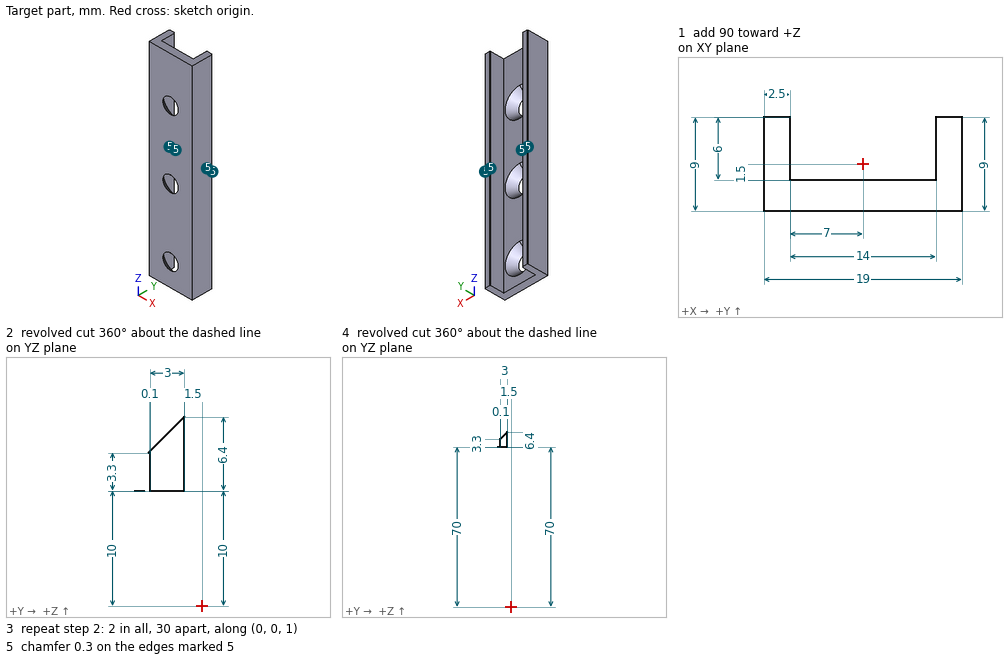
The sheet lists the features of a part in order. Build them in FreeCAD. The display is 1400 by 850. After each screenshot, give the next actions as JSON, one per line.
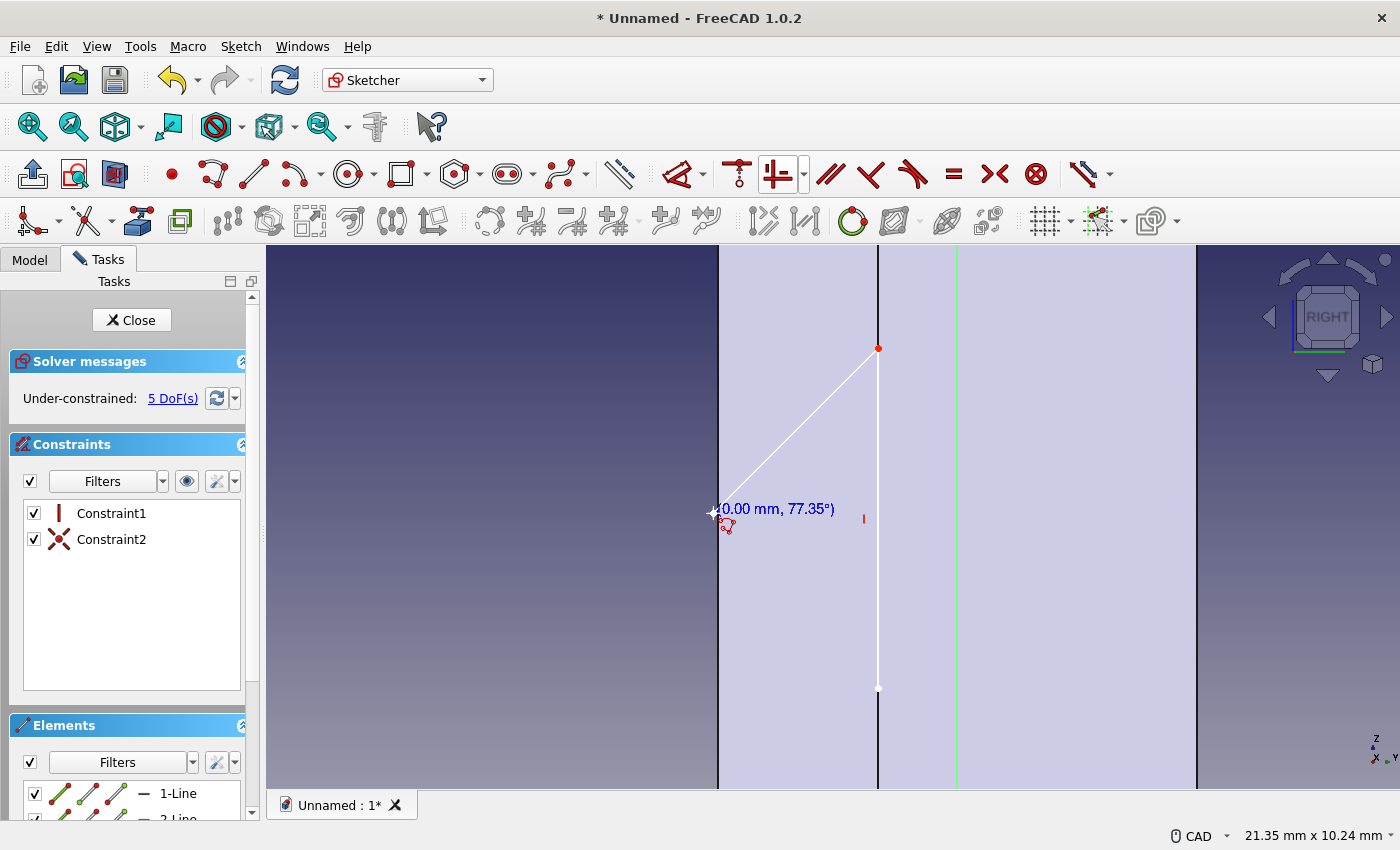
{"action": "scroll", "coordinate": [718, 513], "scroll_direction": "up", "scroll_amount": 8}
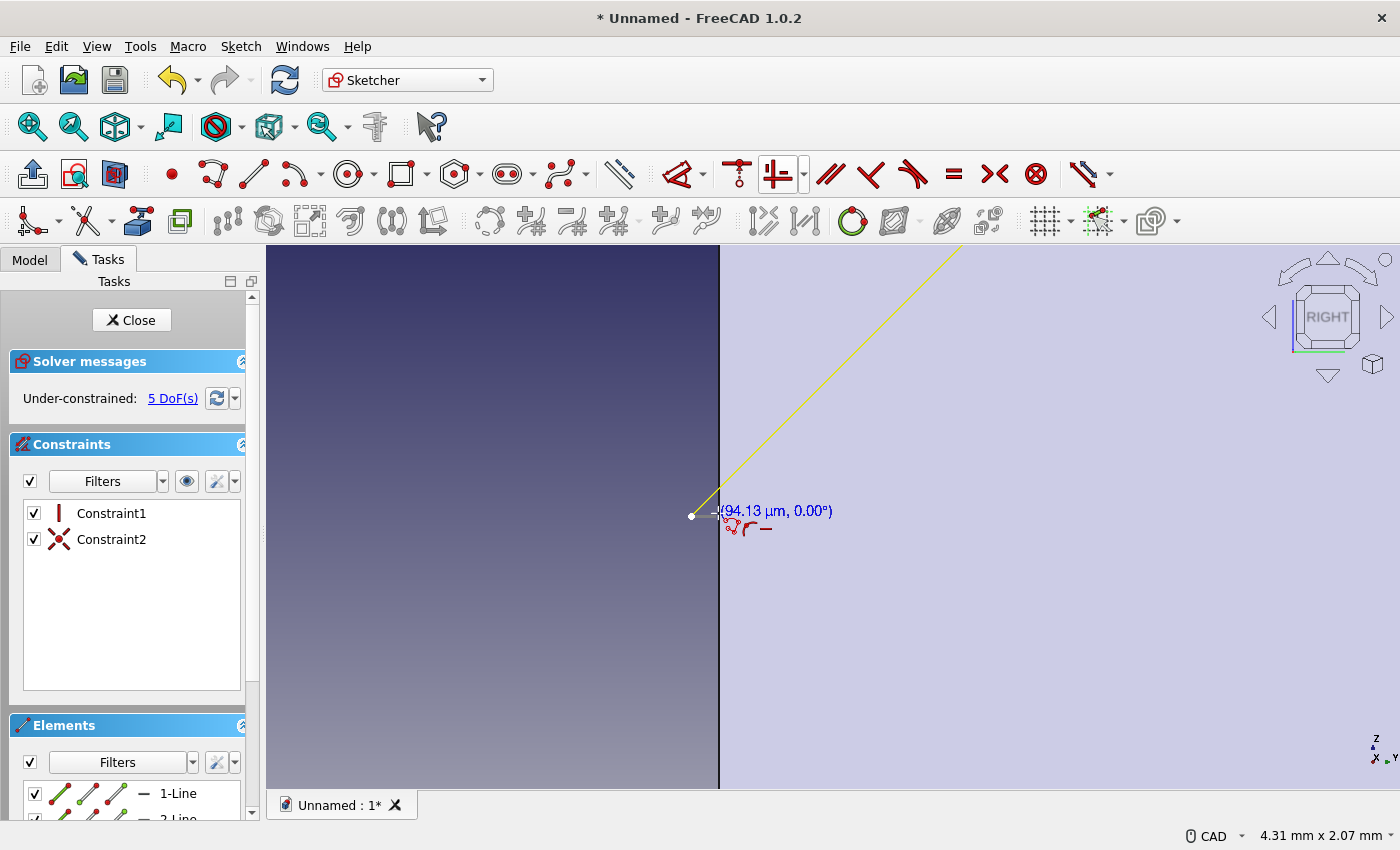
{"action": "left_click", "coordinate": [719, 511]}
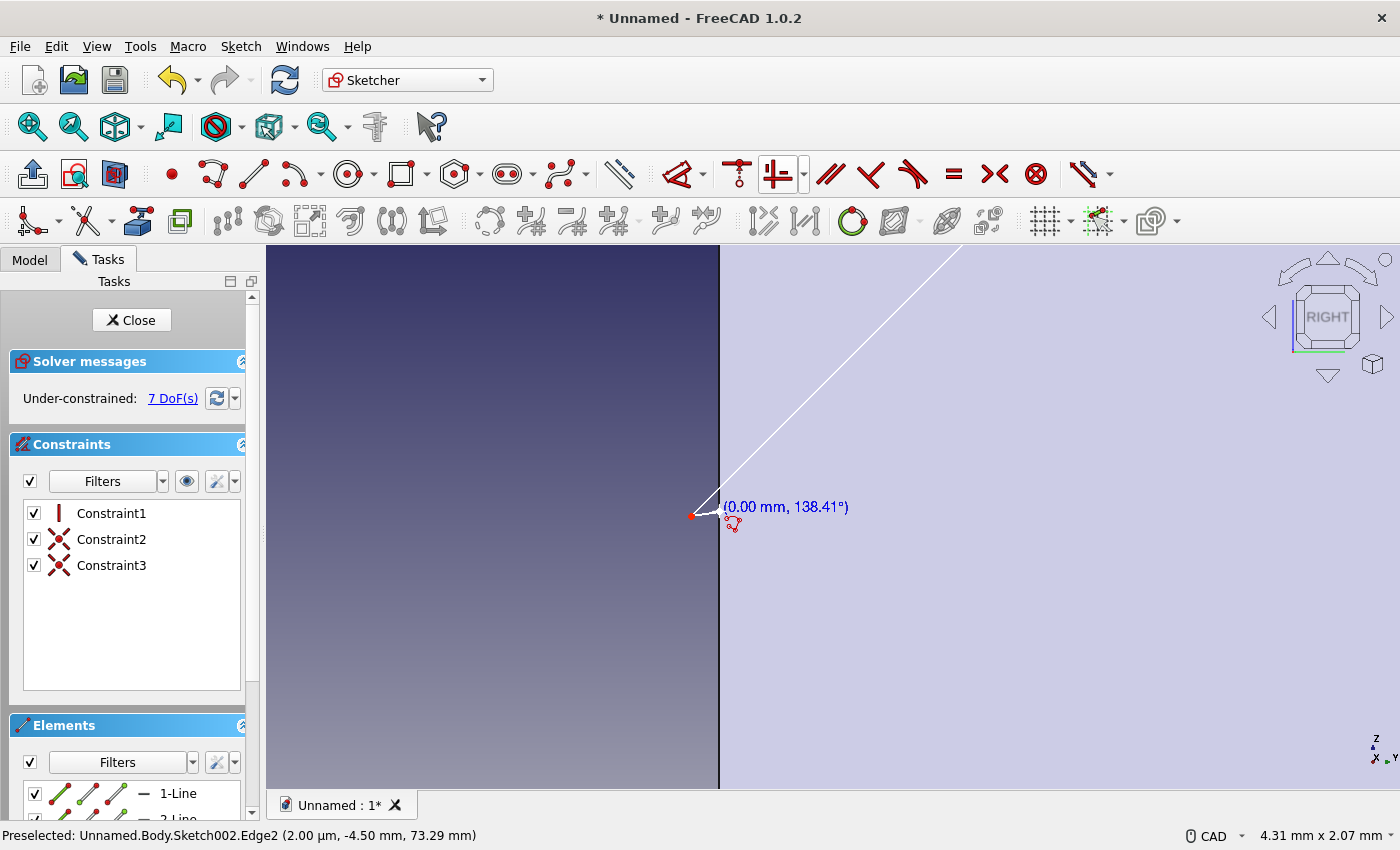
{"action": "scroll", "coordinate": [721, 512], "scroll_direction": "down", "scroll_amount": 8}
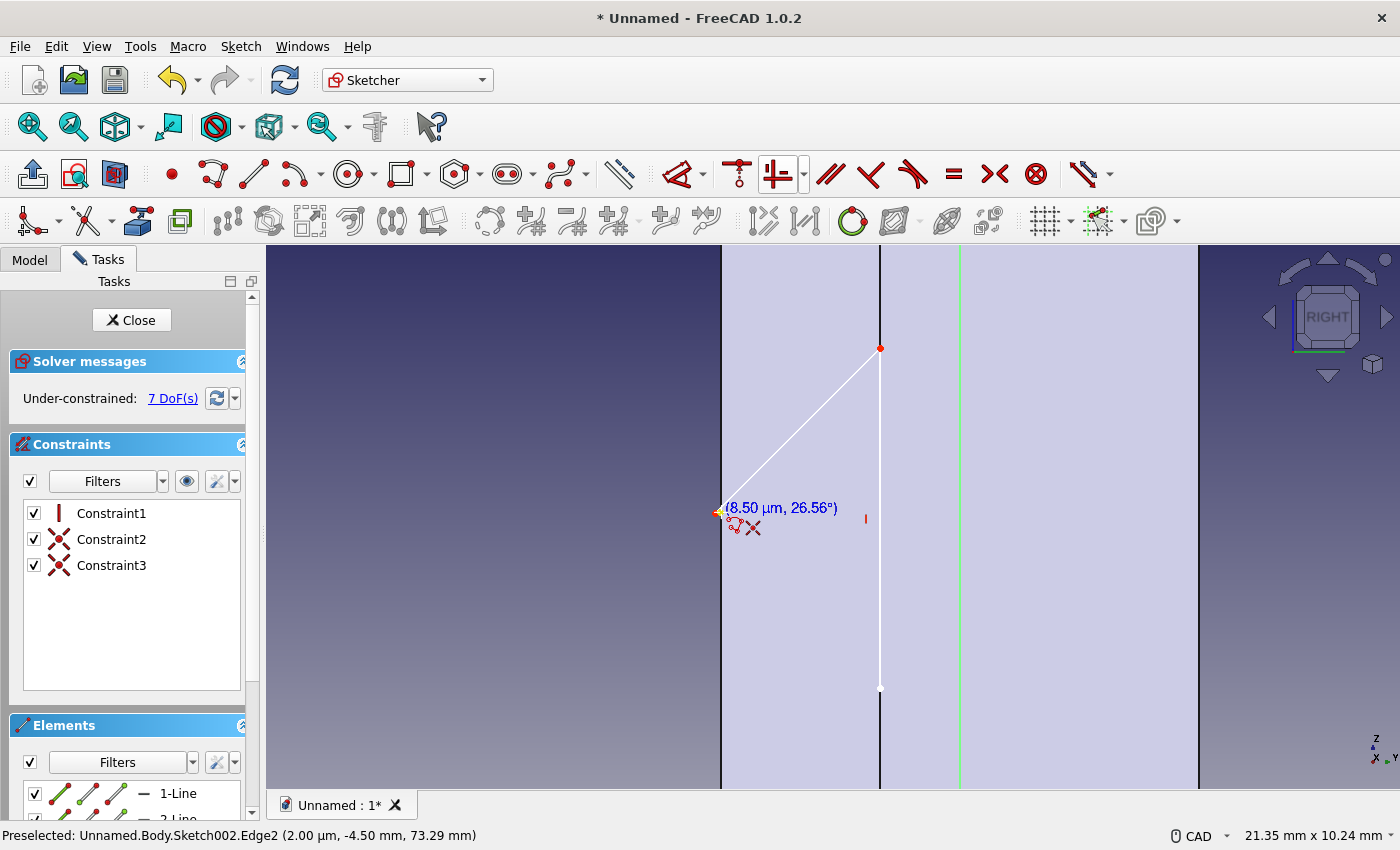
{"action": "left_click", "coordinate": [721, 688]}
{"action": "left_click", "coordinate": [880, 688]}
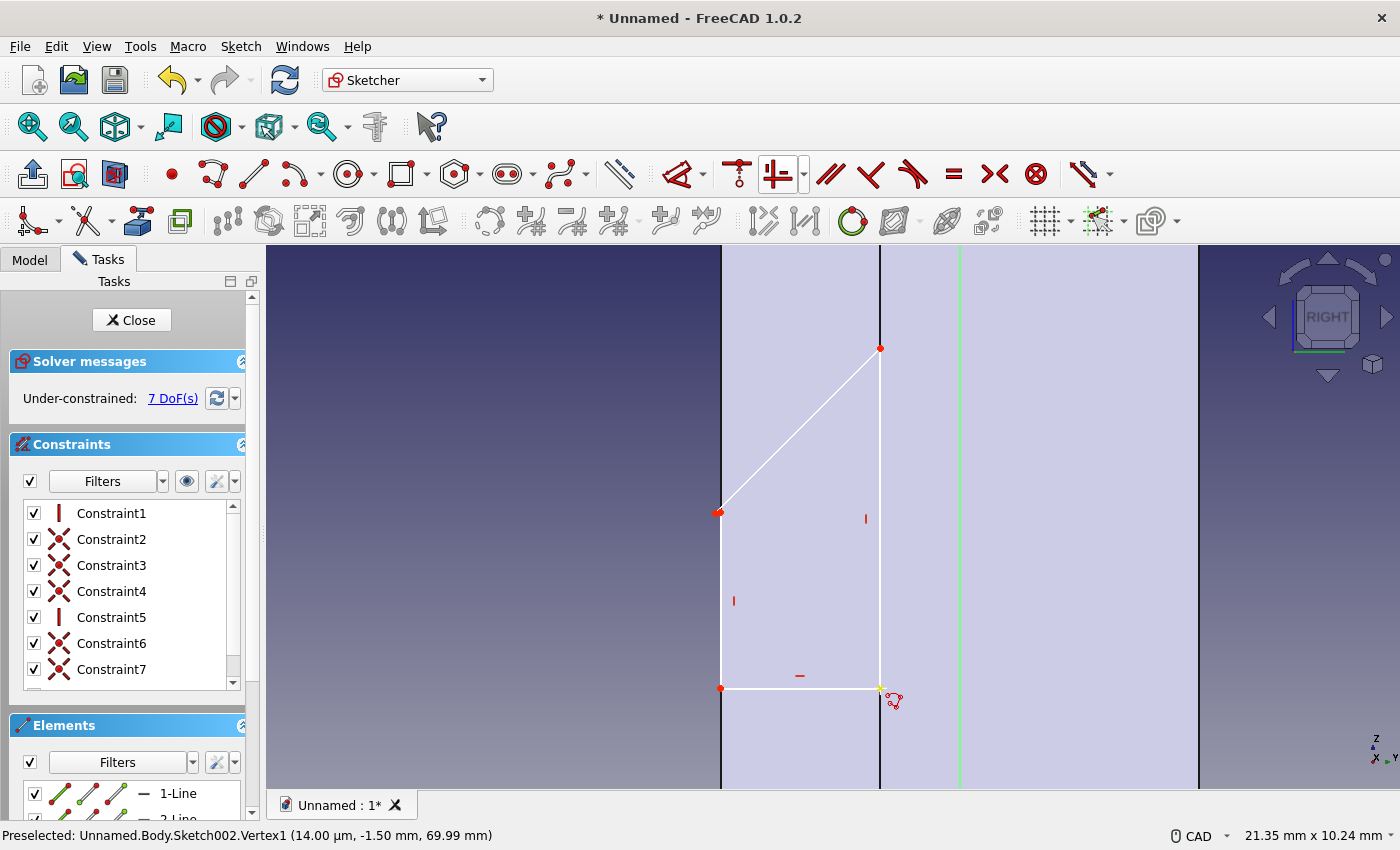
{"action": "key", "text": "g l"}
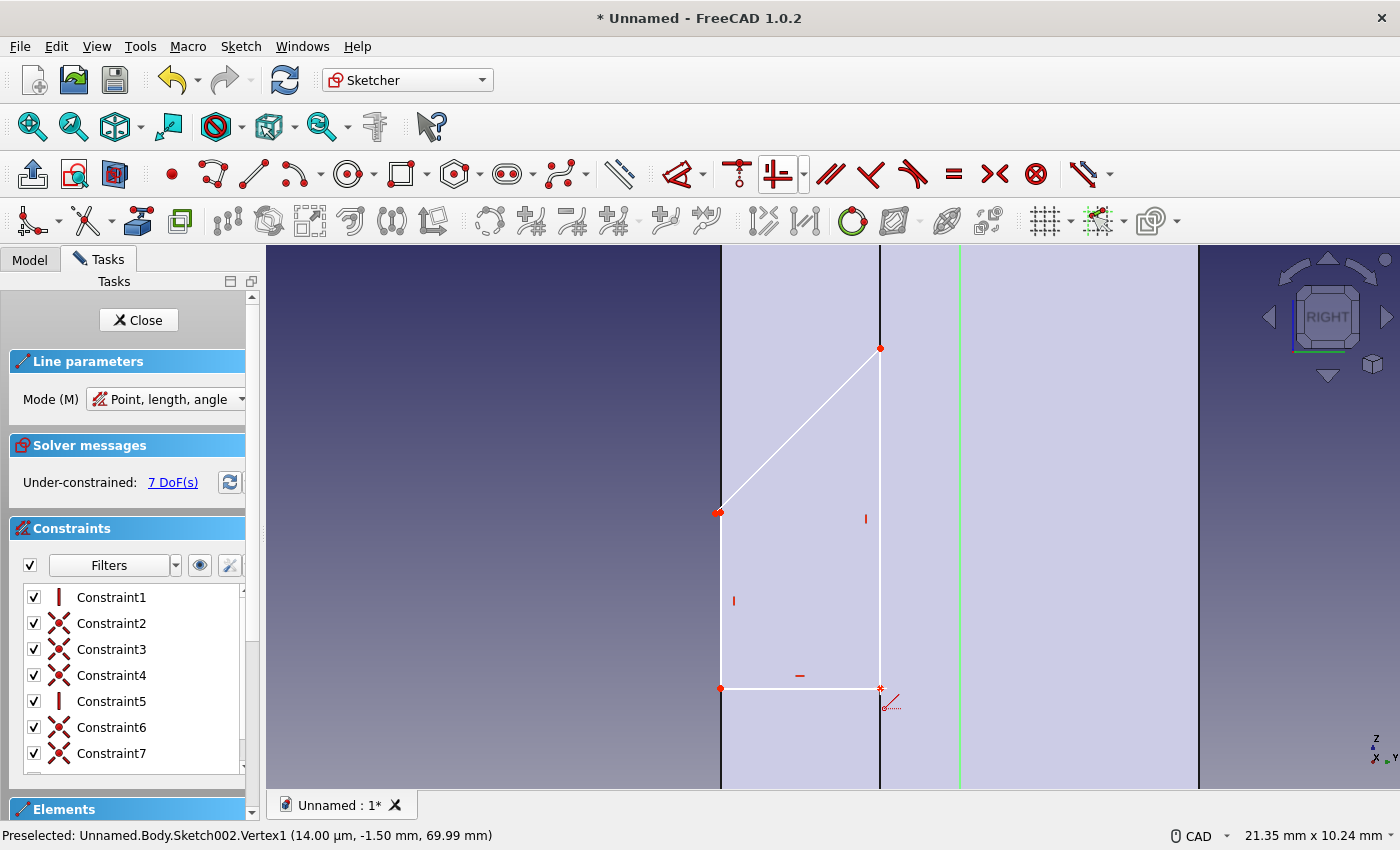
{"action": "left_click", "coordinate": [699, 688]}
{"action": "left_click", "coordinate": [650, 688]}
{"action": "key", "text": "Escape"}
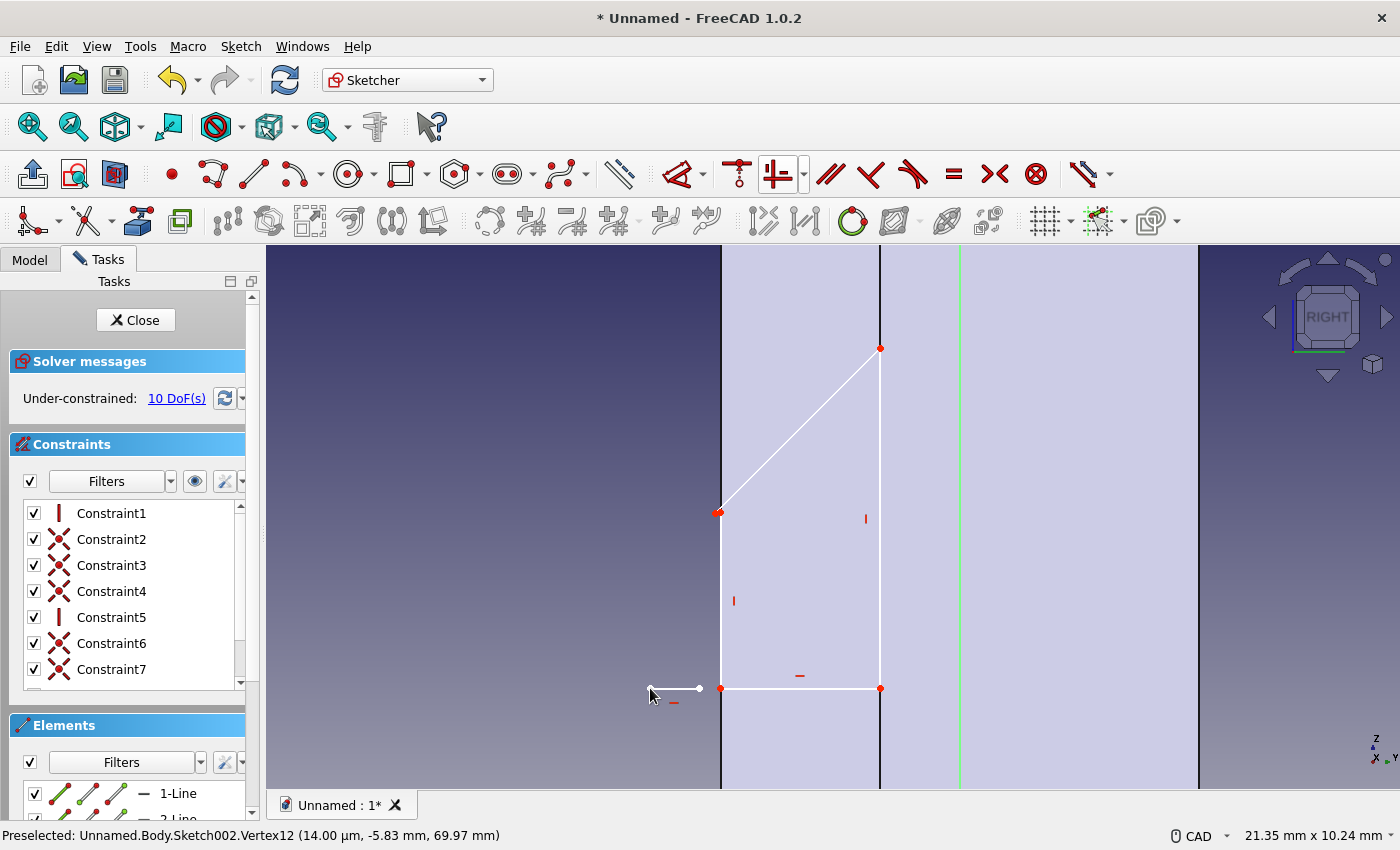
{"action": "left_click", "coordinate": [684, 689]}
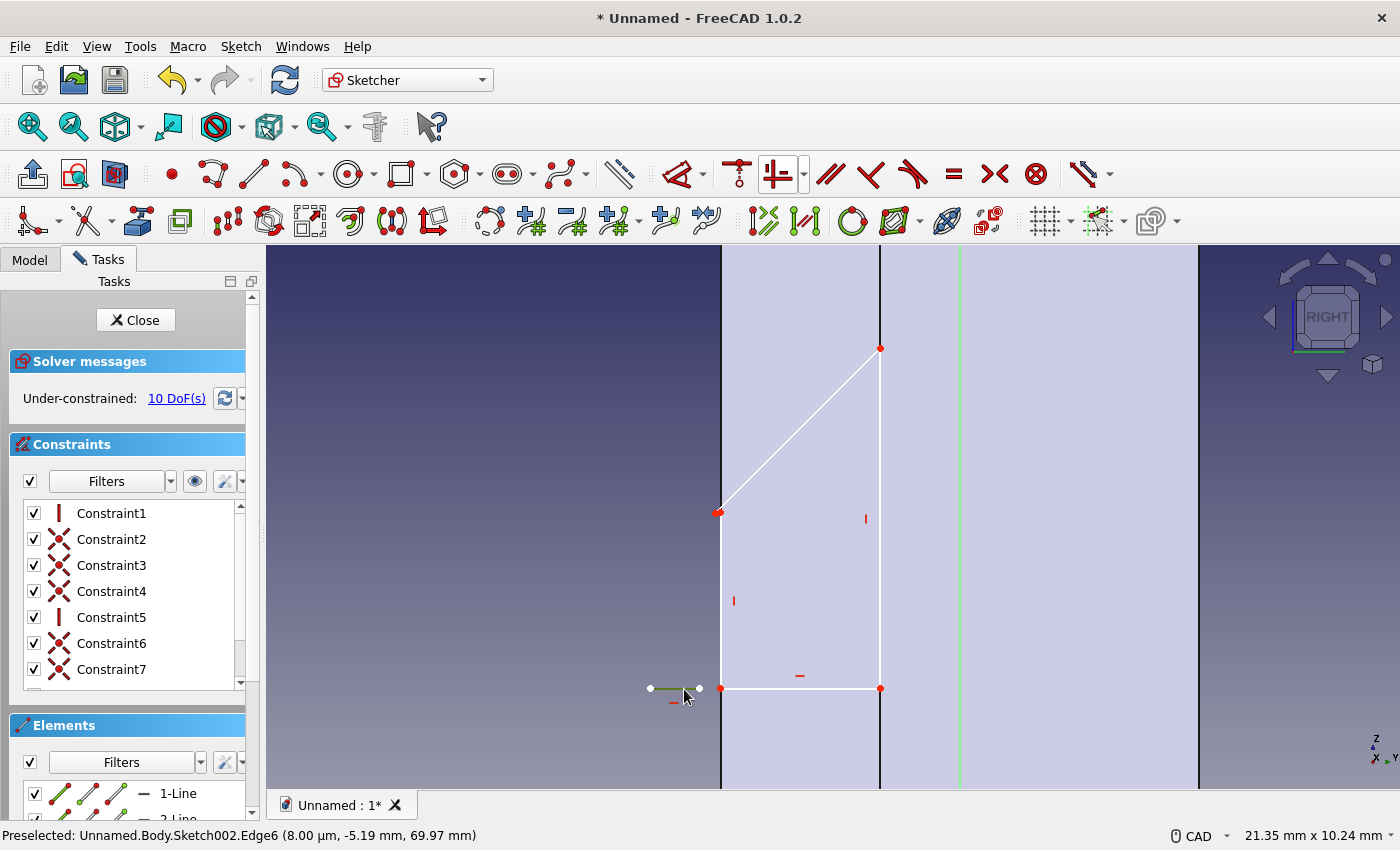
{"action": "left_click", "coordinate": [620, 174]}